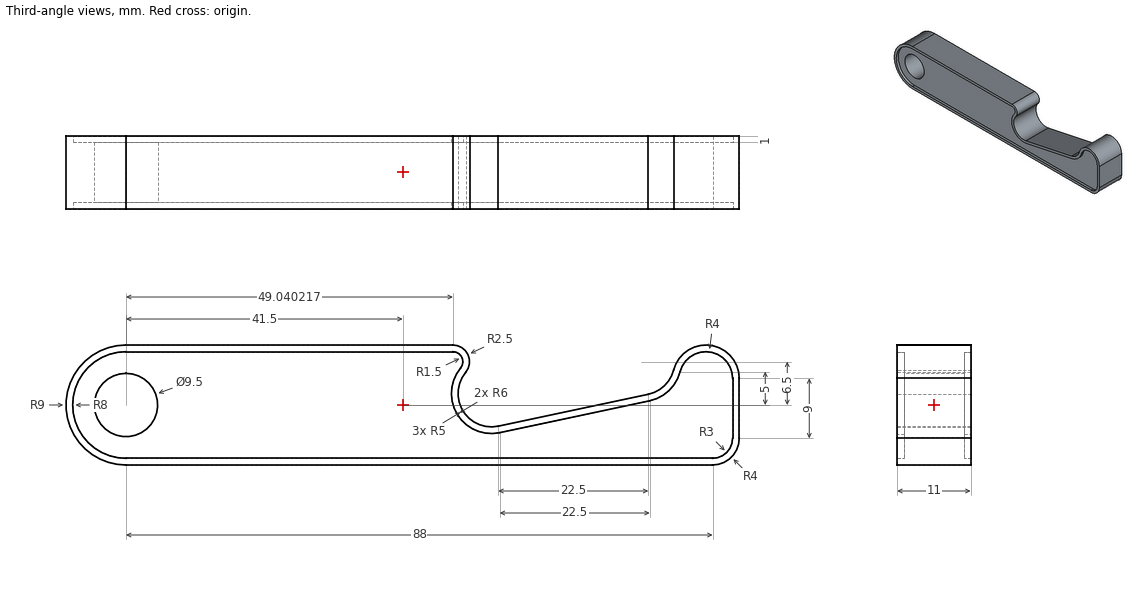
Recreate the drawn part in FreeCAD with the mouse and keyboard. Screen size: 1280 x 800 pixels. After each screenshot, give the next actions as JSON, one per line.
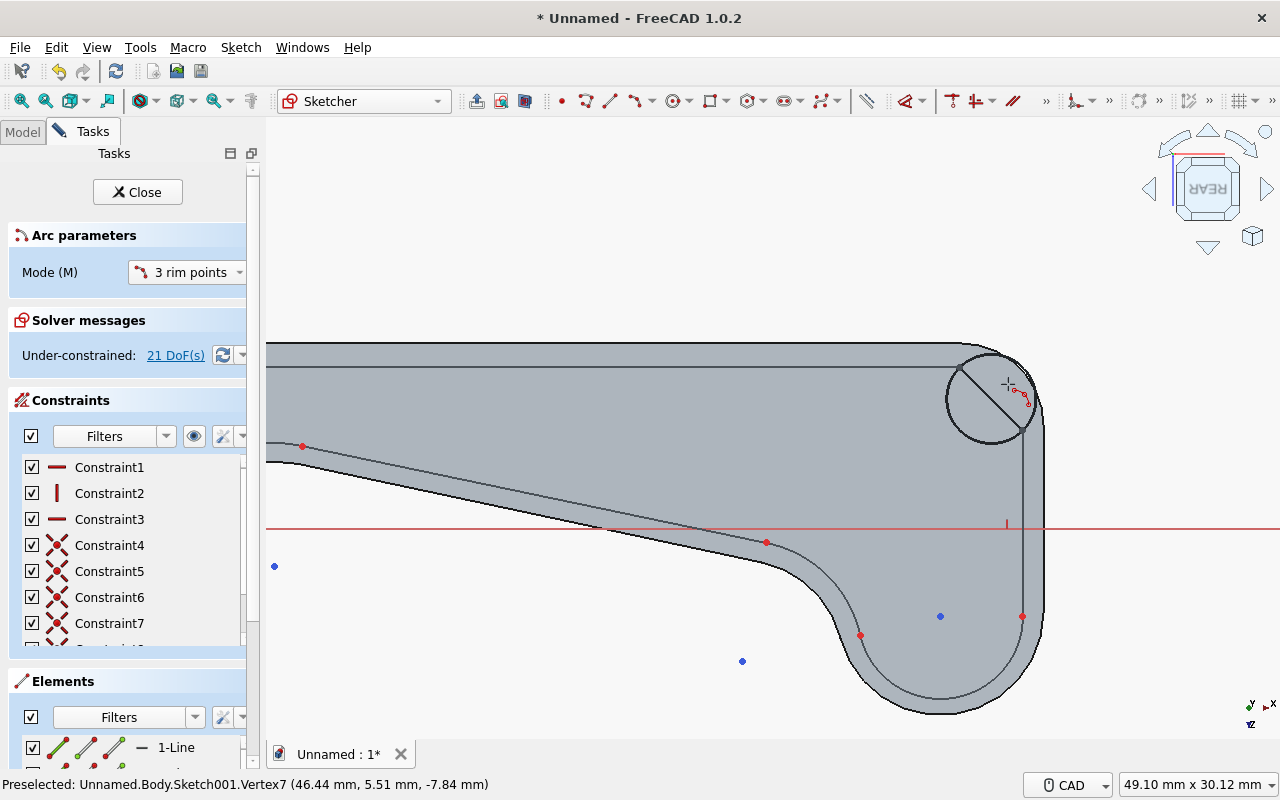
{"action": "left_click", "coordinate": [1005, 382]}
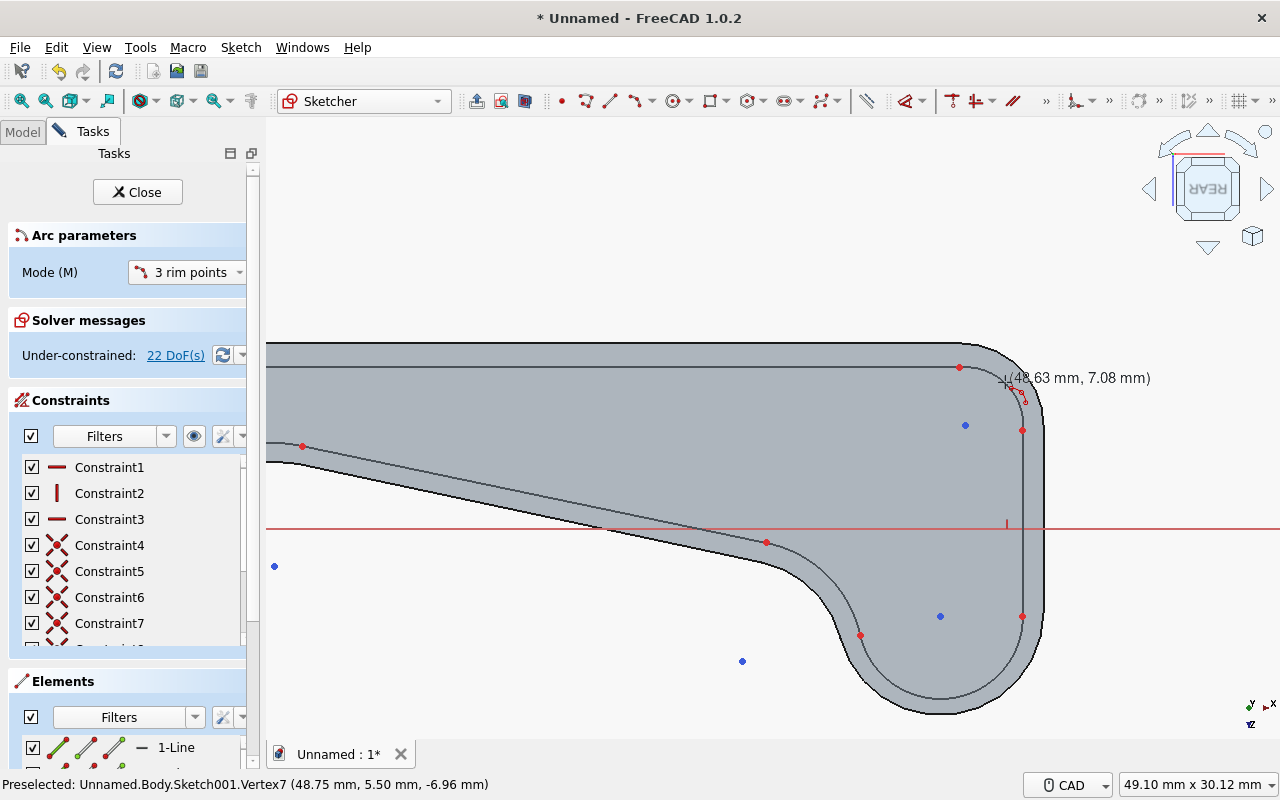
{"action": "scroll", "coordinate": [1008, 384], "scroll_direction": "down", "scroll_amount": 6}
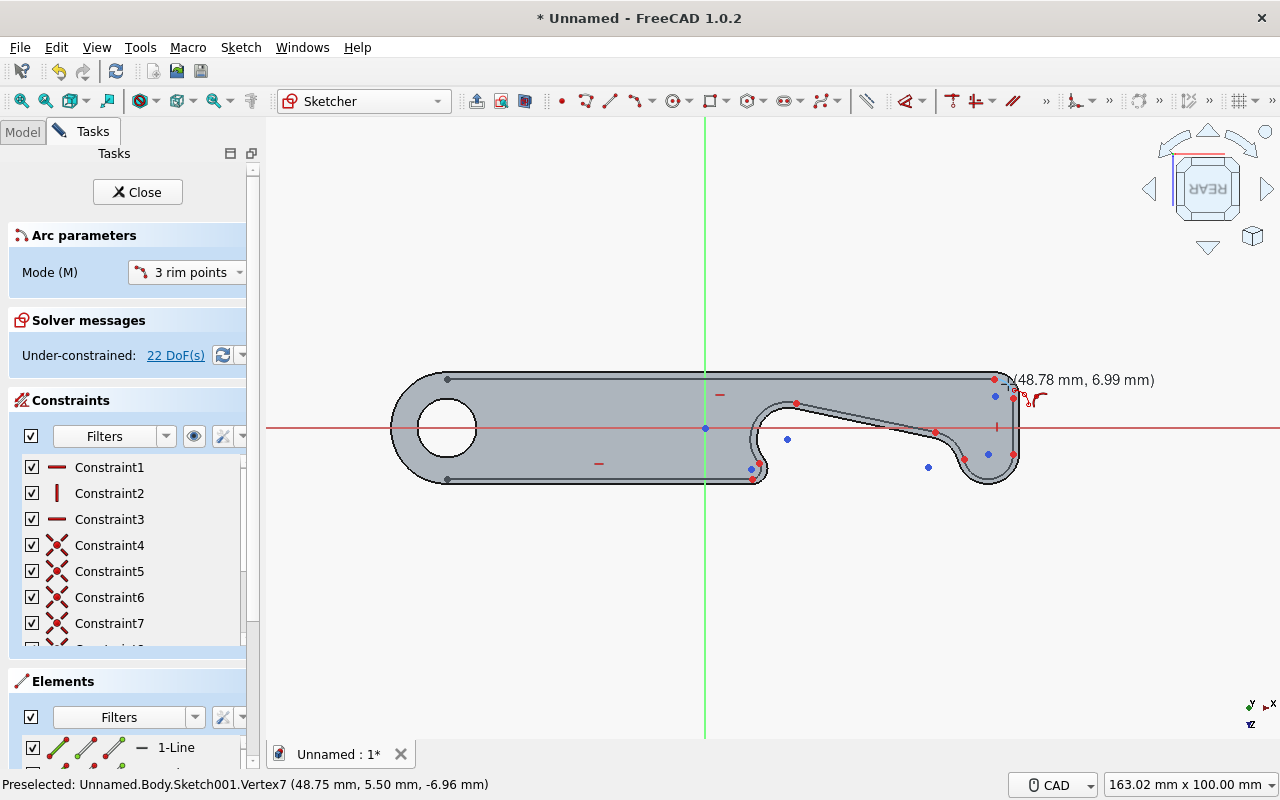
{"action": "left_click", "coordinate": [447, 379]}
{"action": "left_click", "coordinate": [447, 479]}
{"action": "left_click", "coordinate": [400, 413]}
{"action": "key", "text": "Escape"}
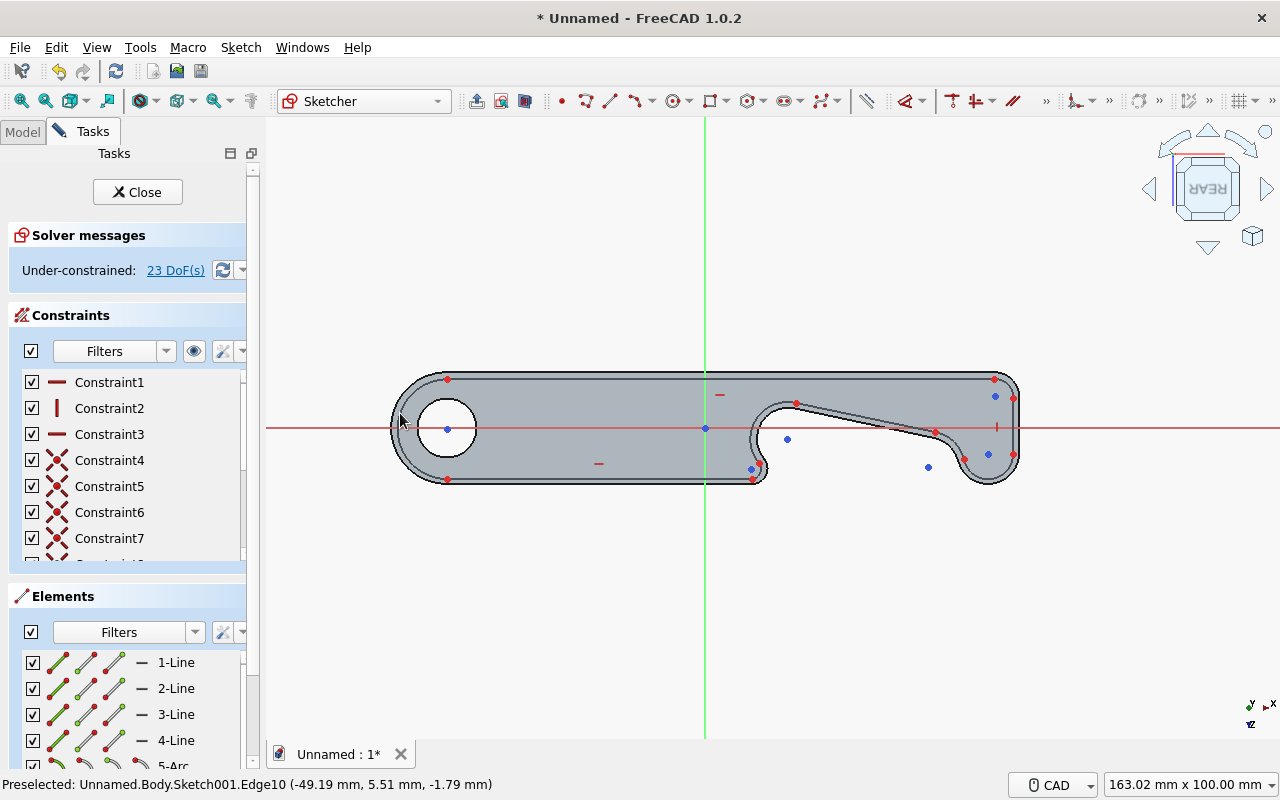
{"action": "left_click", "coordinate": [539, 479]}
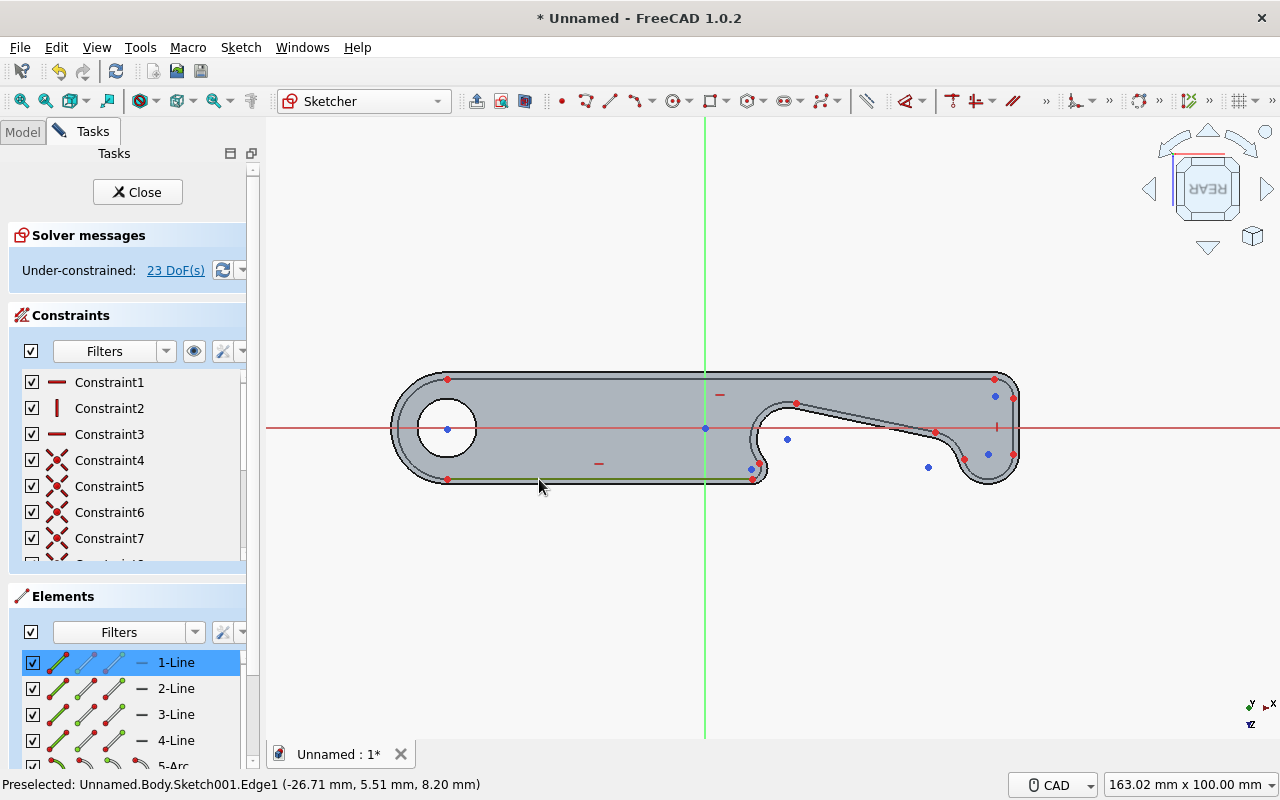
{"action": "scroll", "coordinate": [760, 473], "scroll_direction": "up", "scroll_amount": 2}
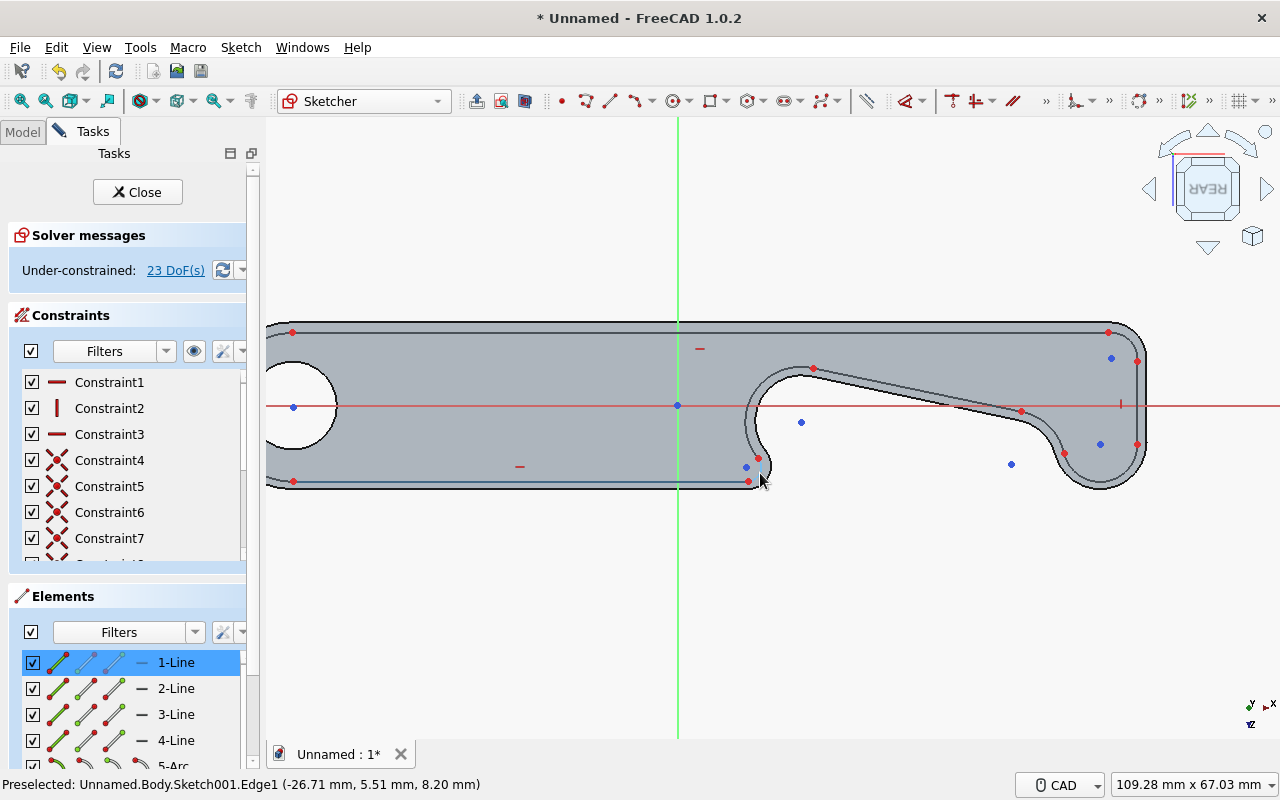
{"action": "left_click", "coordinate": [760, 473]}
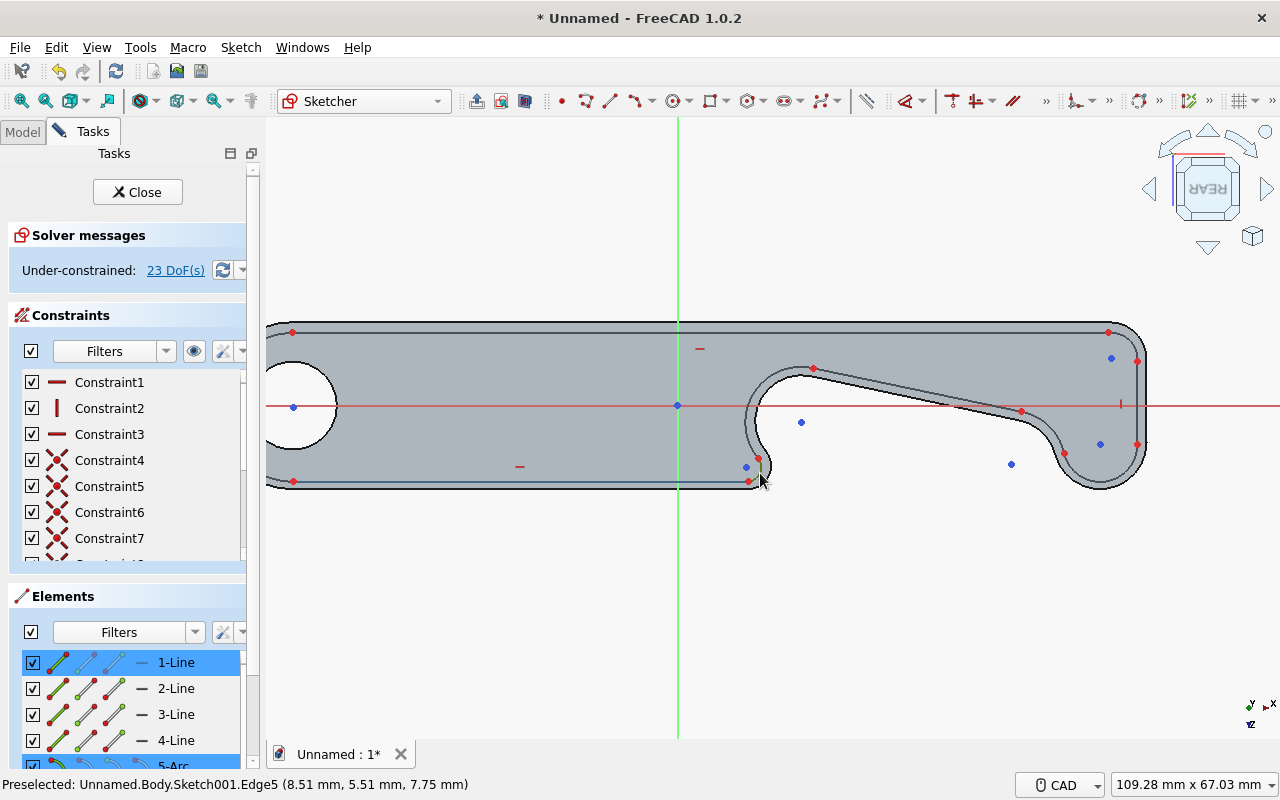
{"action": "key", "text": "t"}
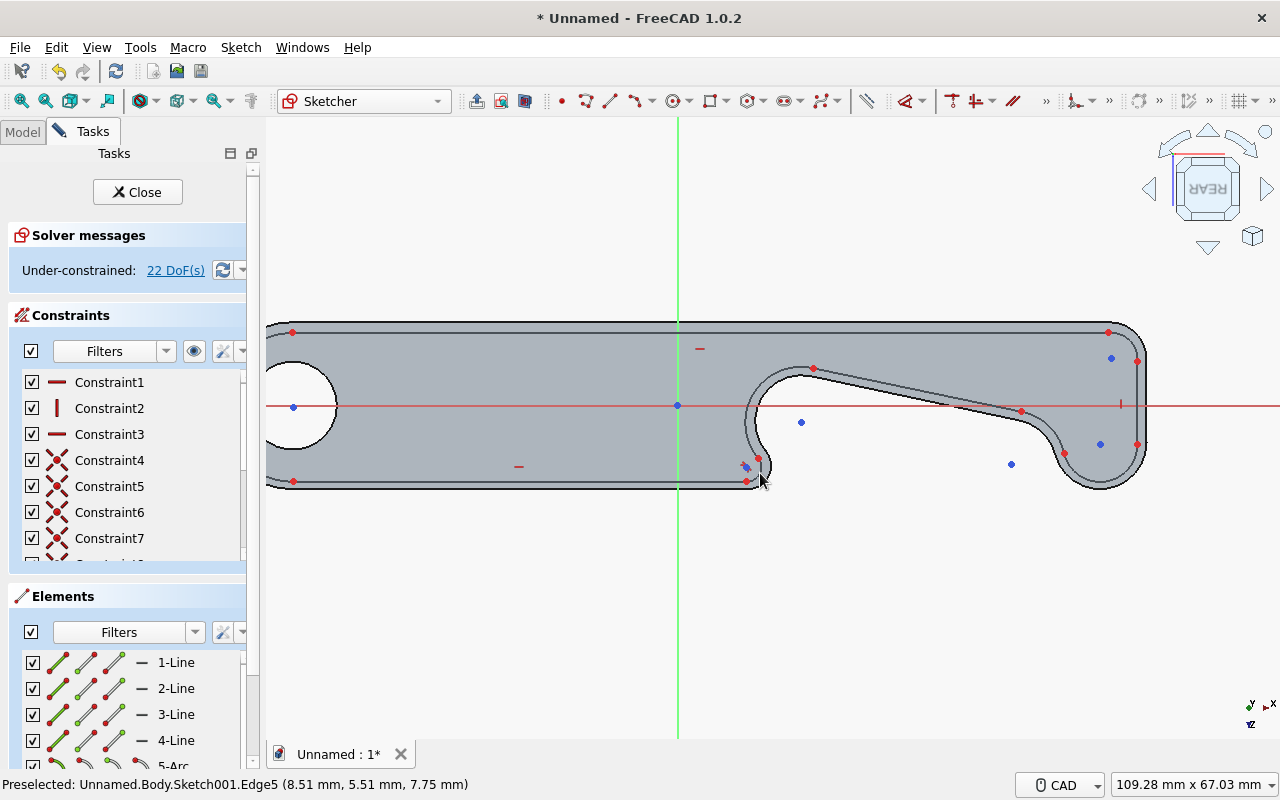
{"action": "left_click", "coordinate": [429, 482]}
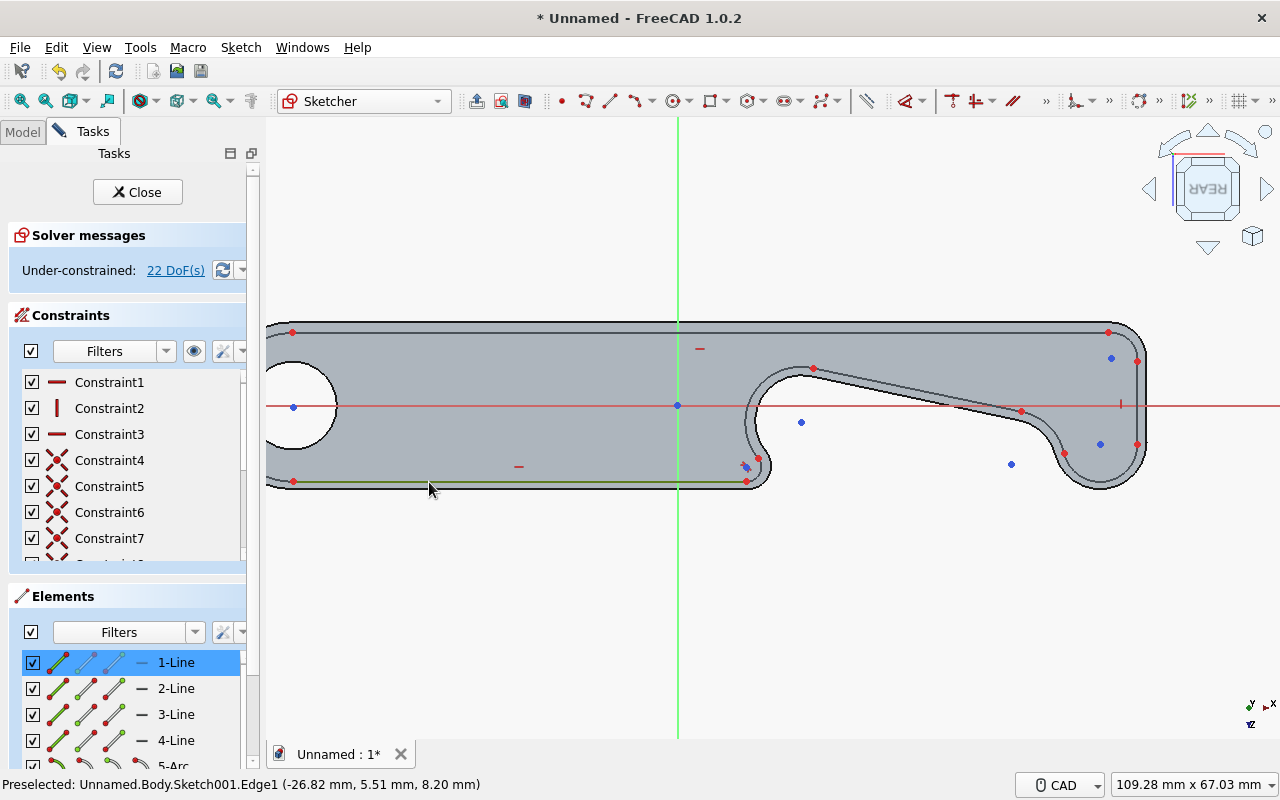
{"action": "scroll", "coordinate": [759, 473], "scroll_direction": "down", "scroll_amount": 2}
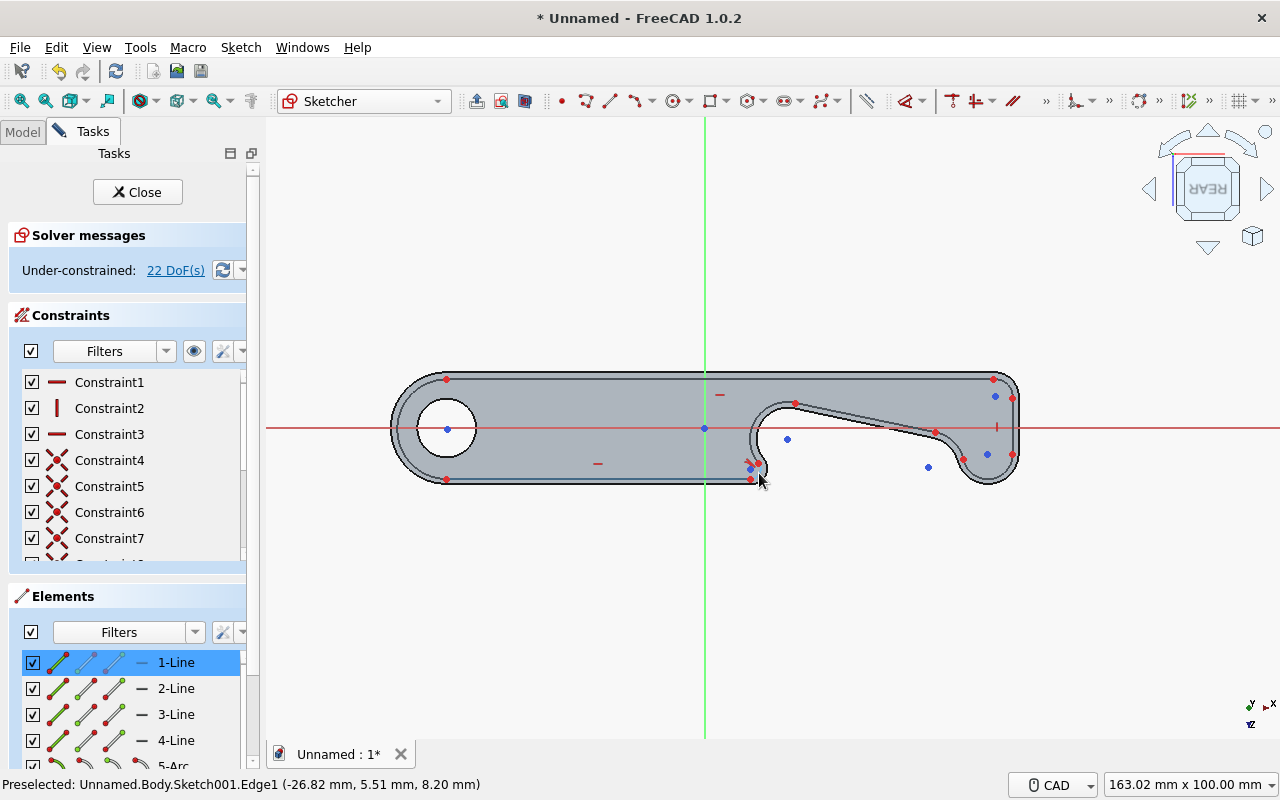
{"action": "left_click", "coordinate": [407, 400]}